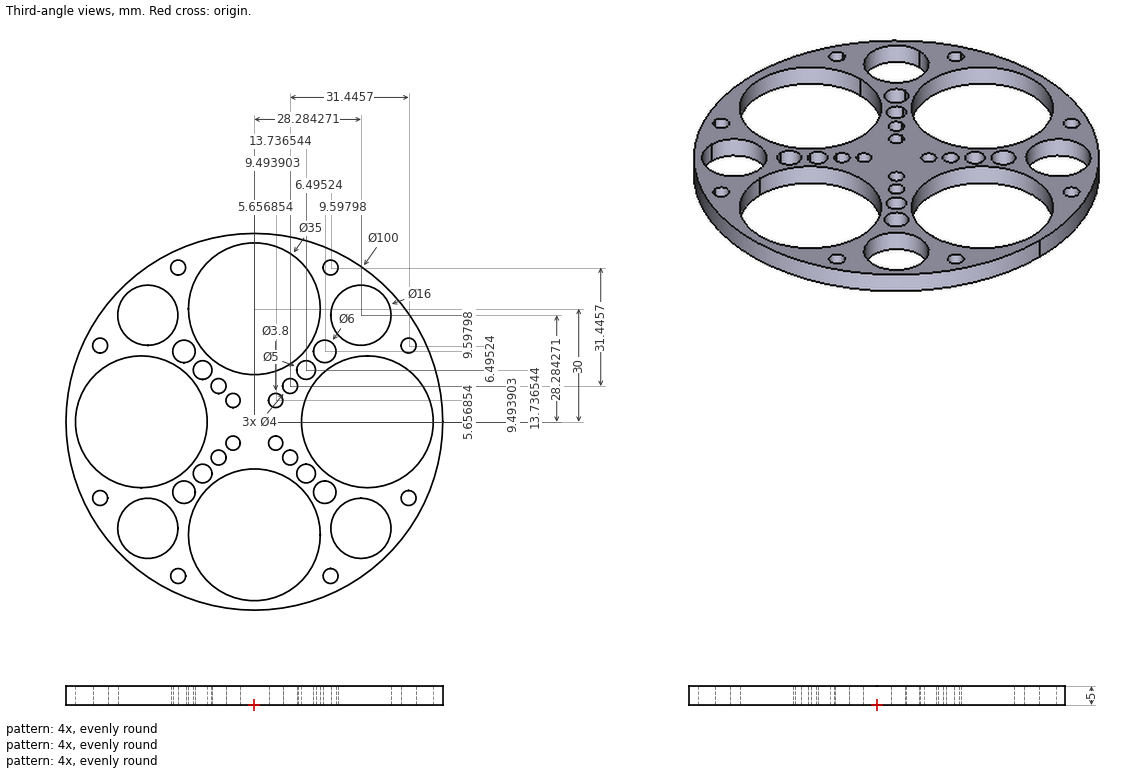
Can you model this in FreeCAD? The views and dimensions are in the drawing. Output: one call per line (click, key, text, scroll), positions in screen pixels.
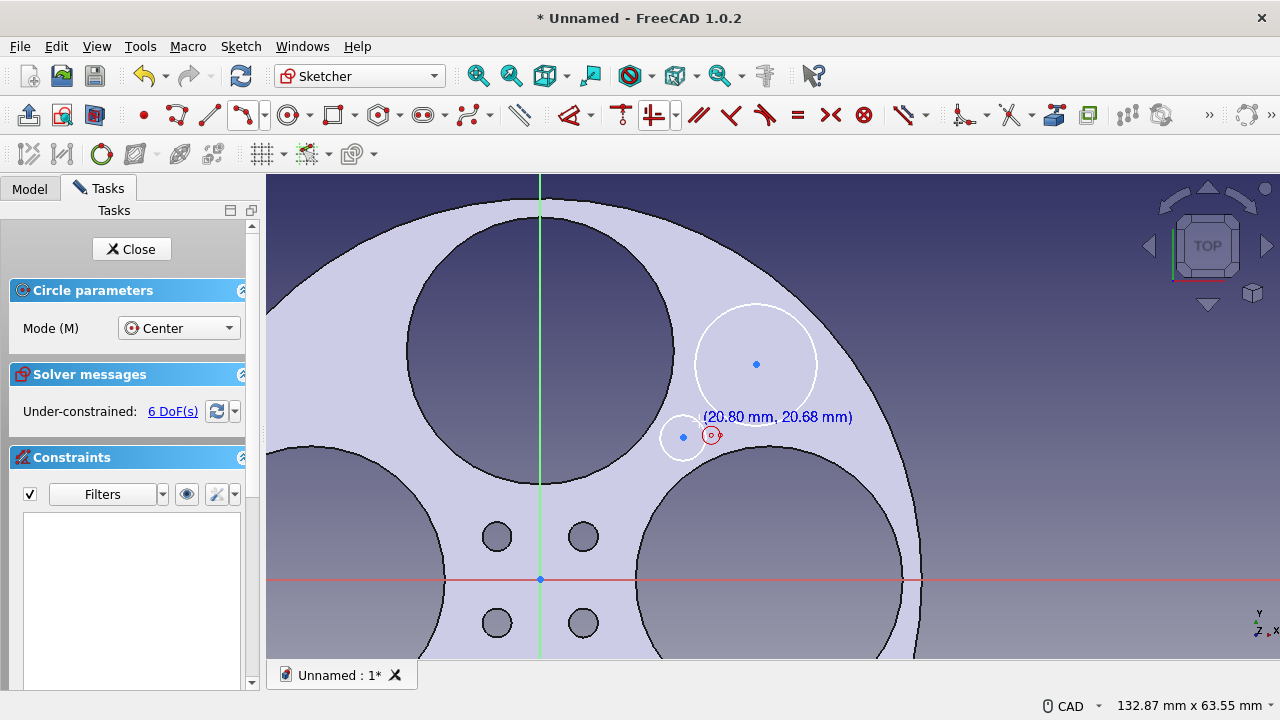
click(645, 475)
click(632, 462)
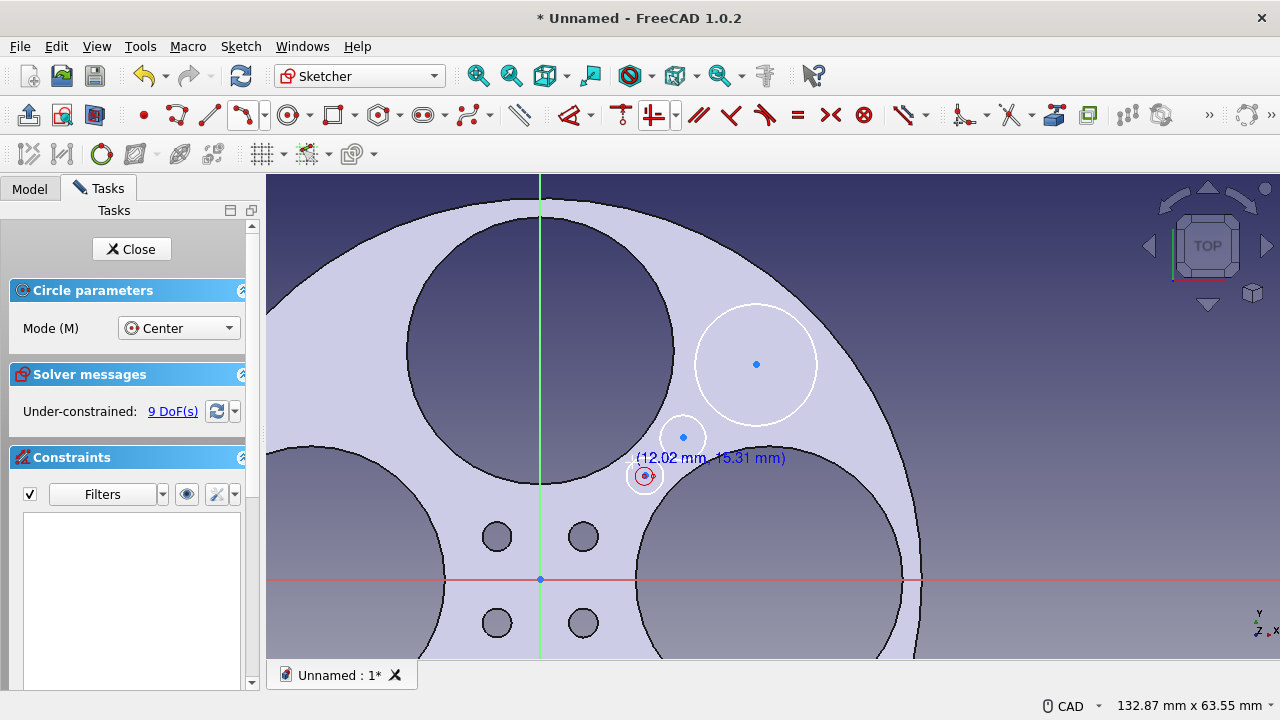
scroll(613, 507, up, 2)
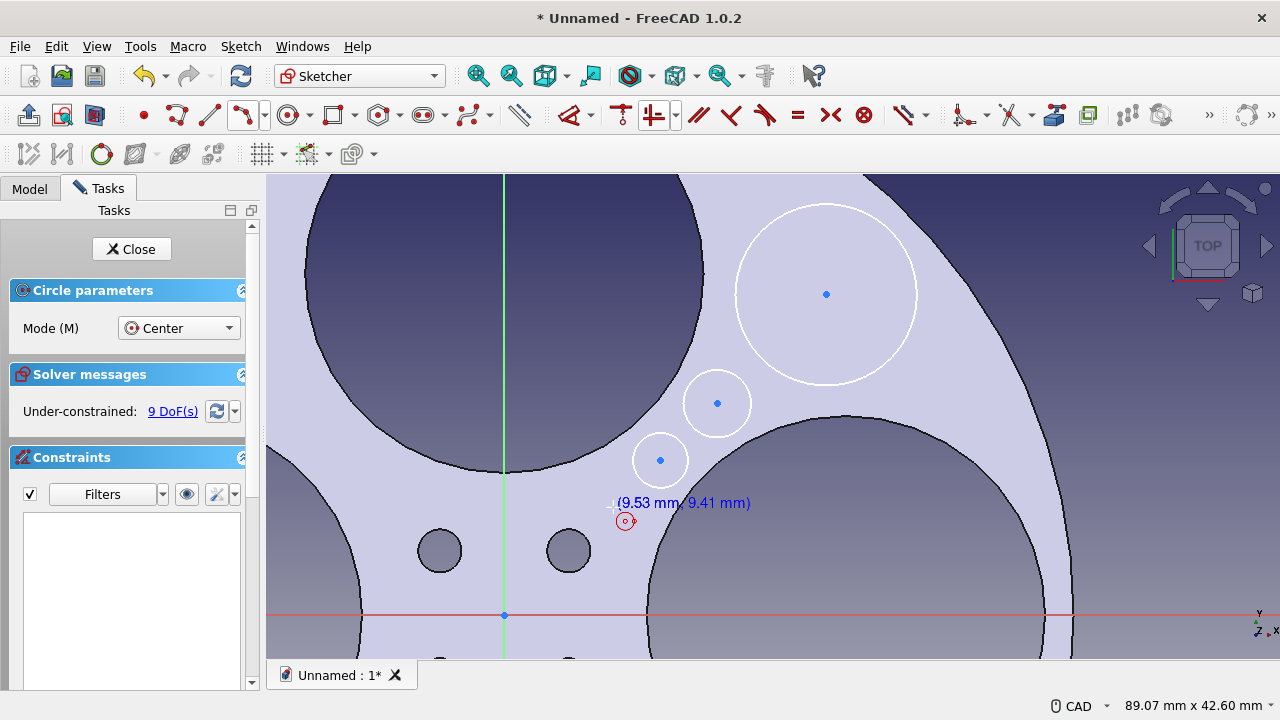
click(612, 507)
click(629, 491)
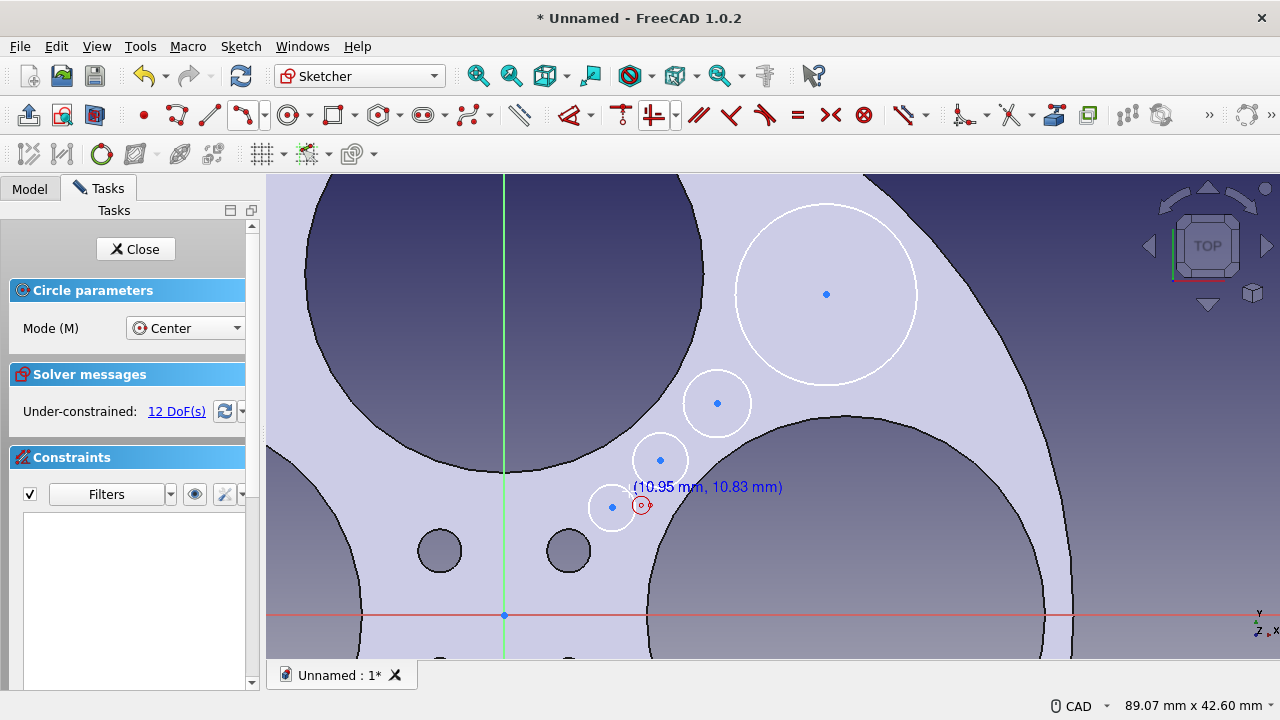
scroll(614, 509, down, 2)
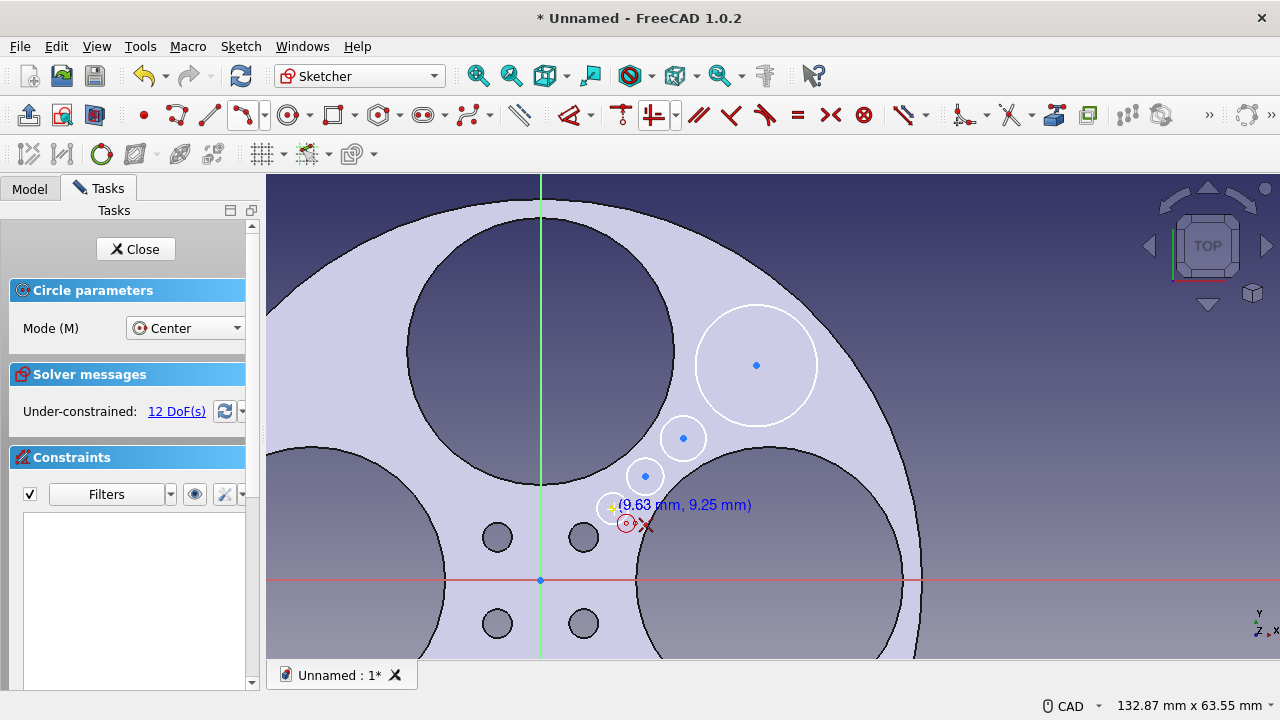
scroll(695, 268, up, 2)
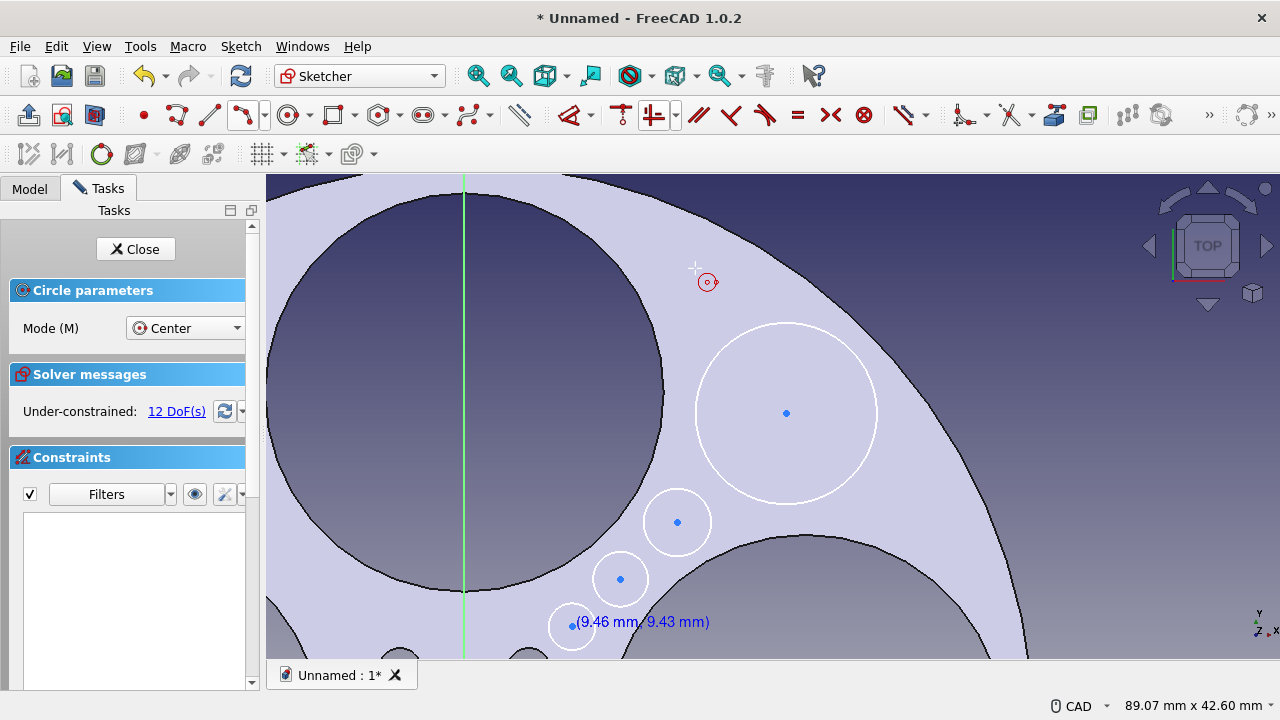
click(695, 268)
click(711, 252)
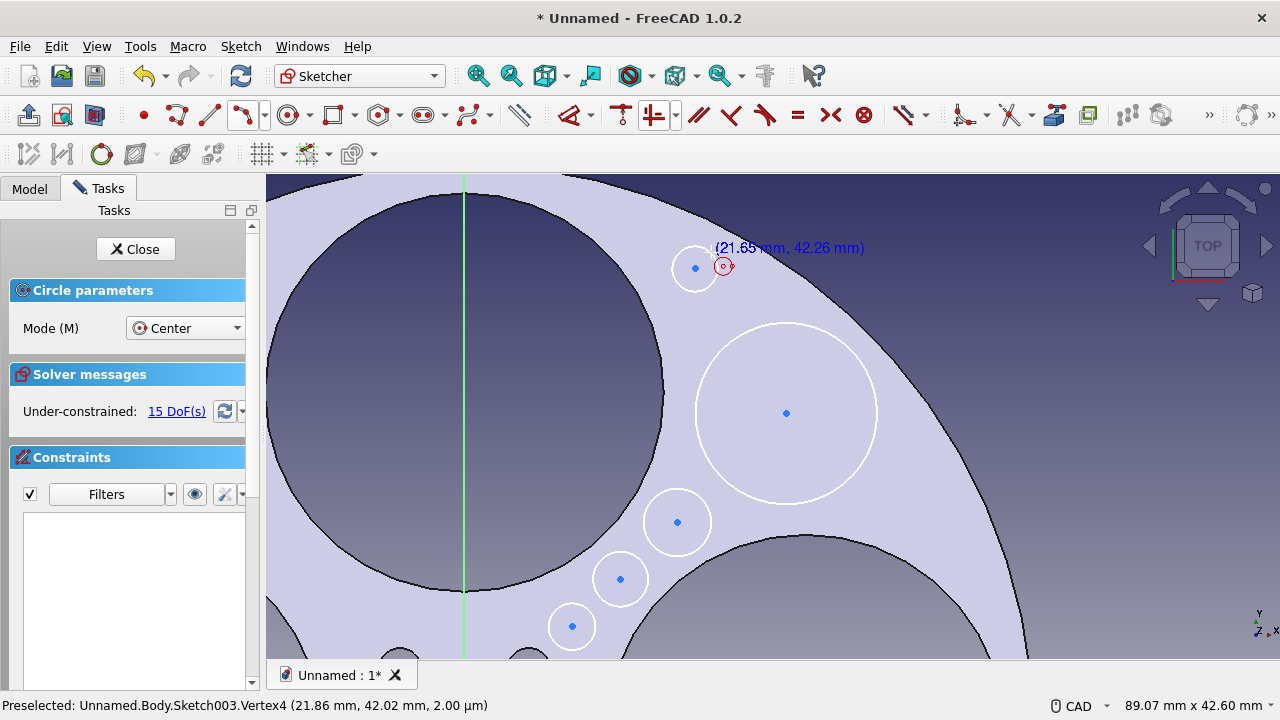
click(931, 504)
click(947, 488)
key(Escape)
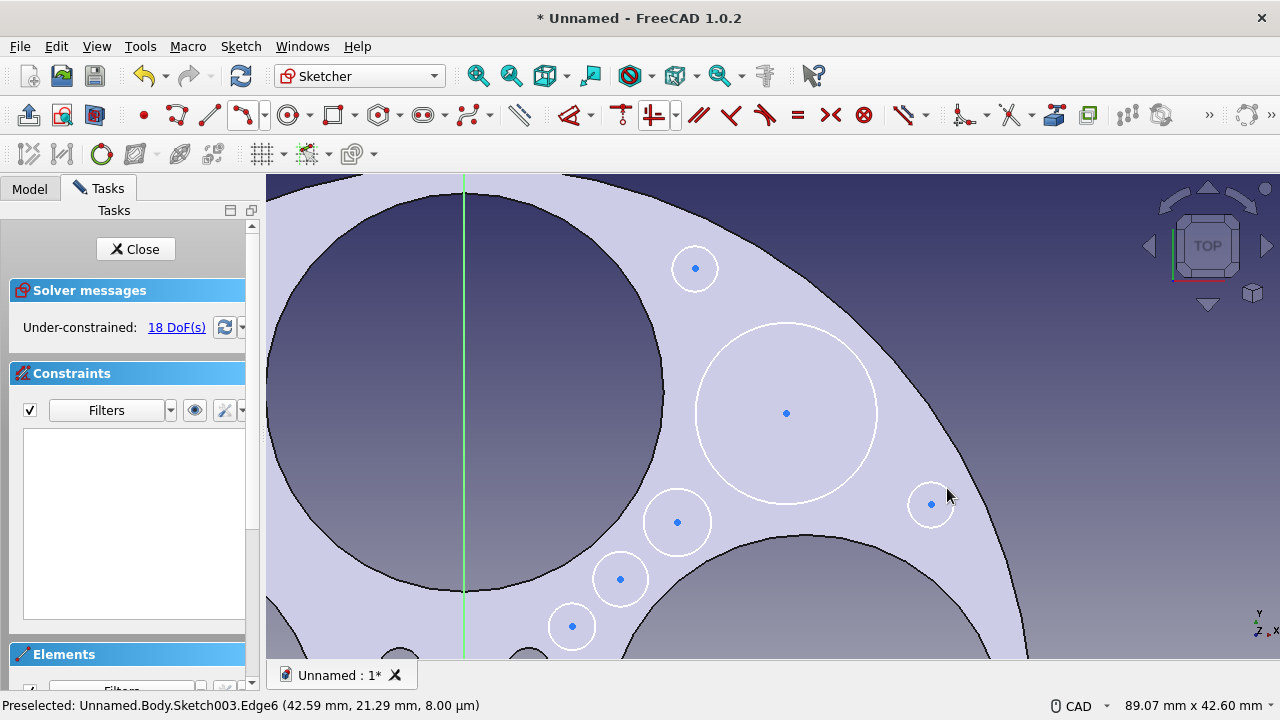
click(589, 610)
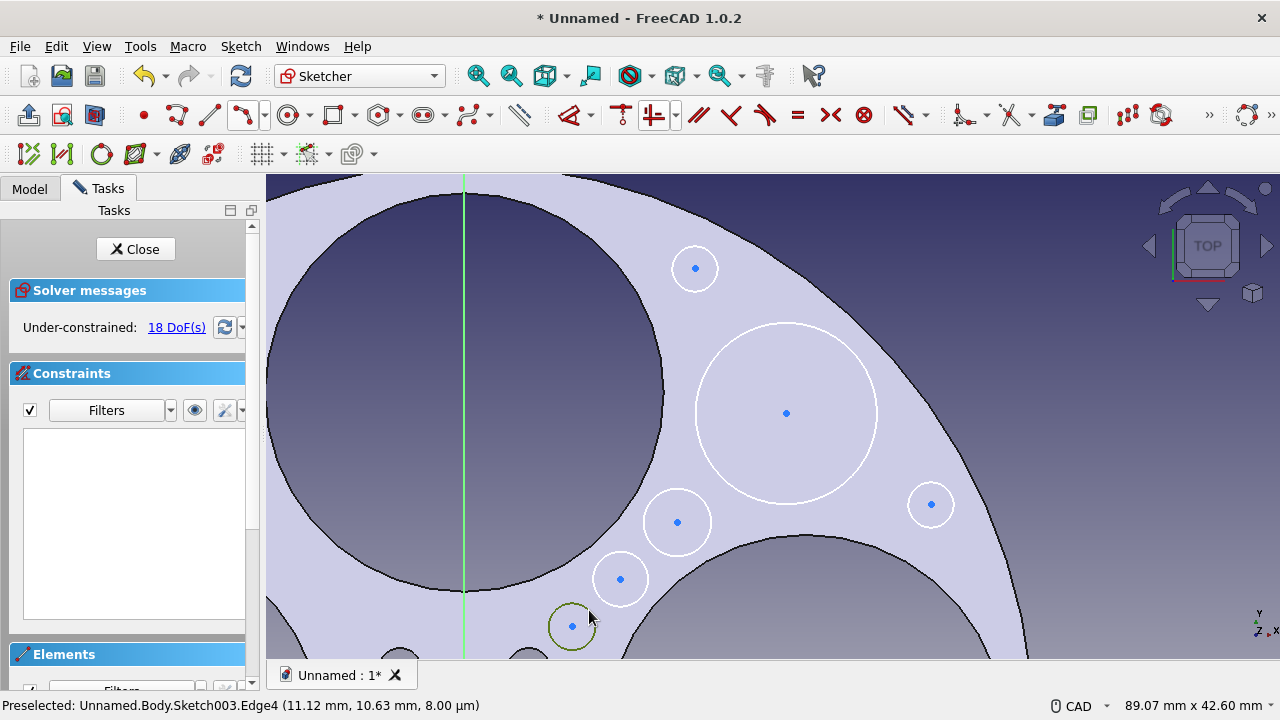
click(711, 253)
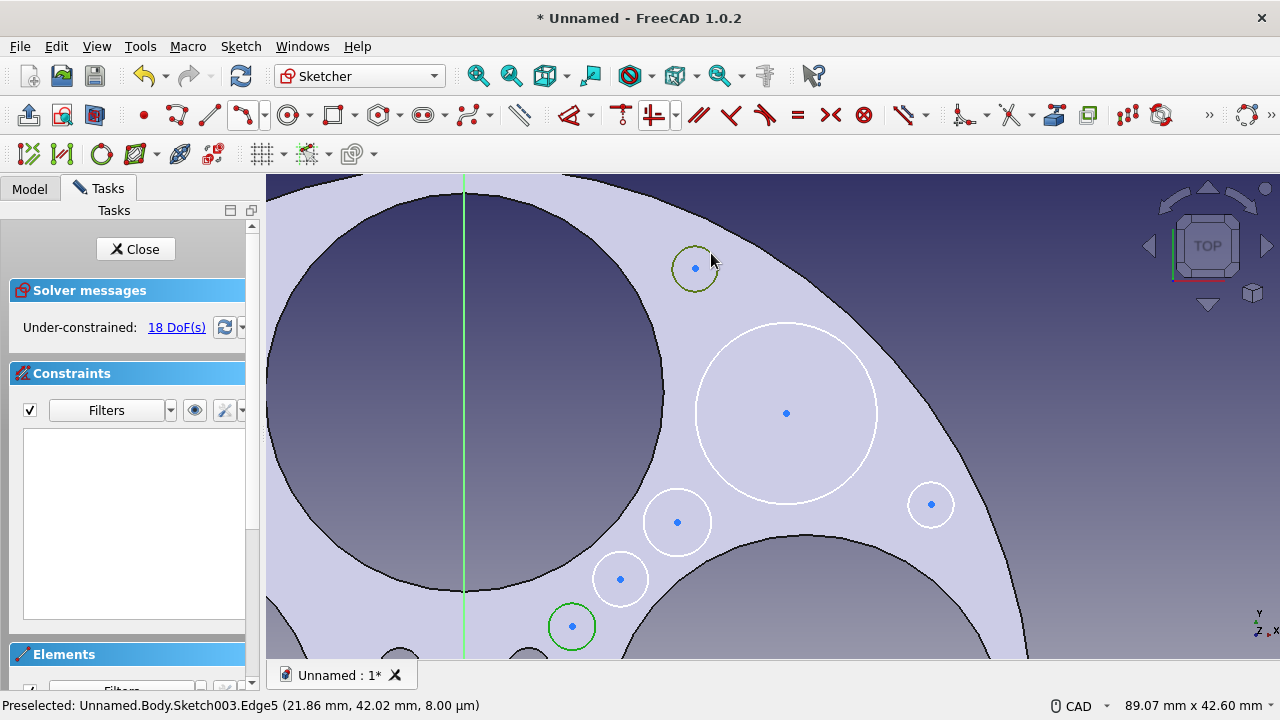
click(947, 489)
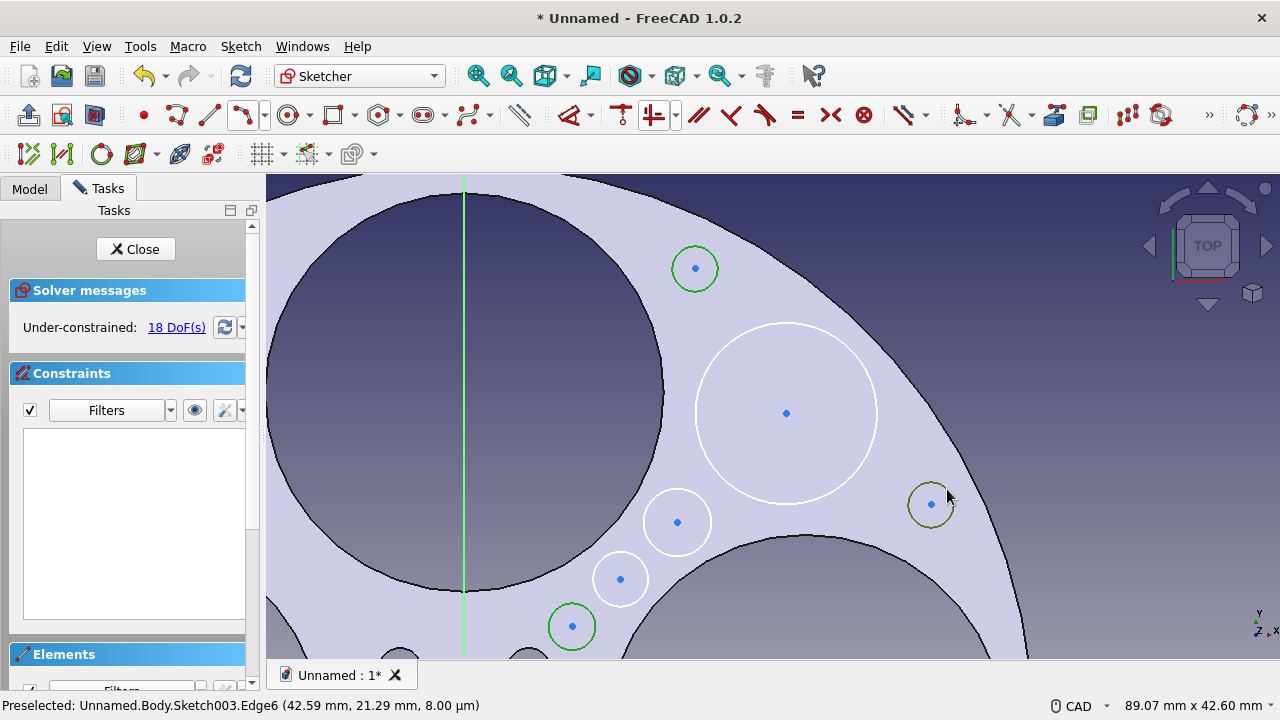
click(798, 116)